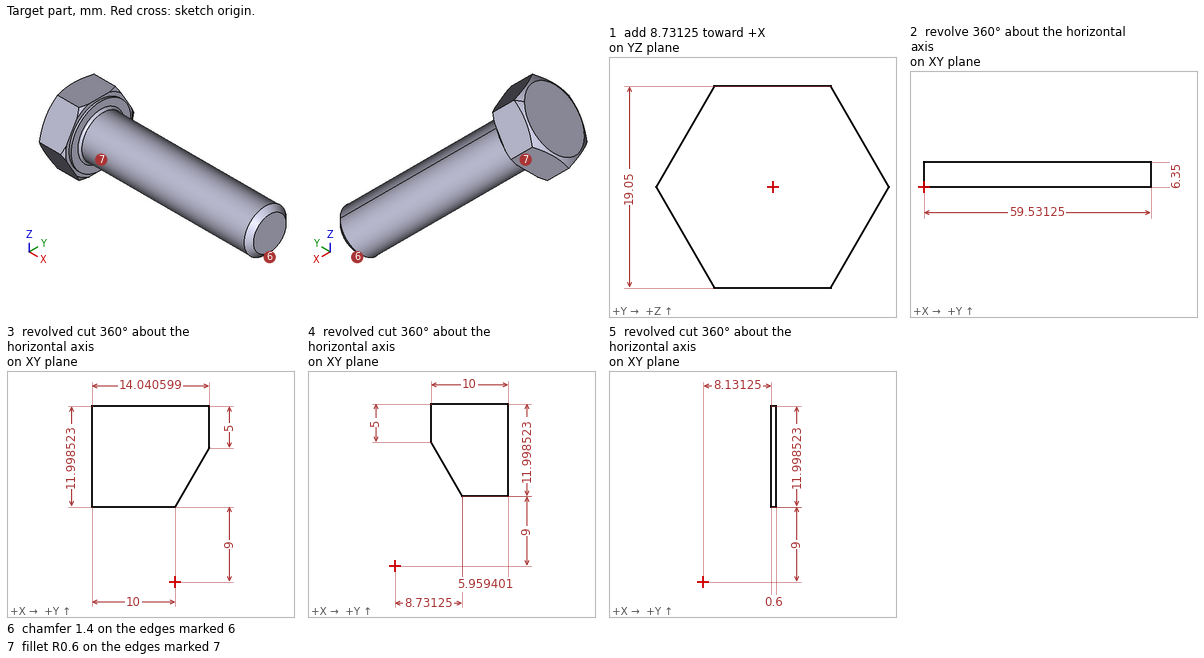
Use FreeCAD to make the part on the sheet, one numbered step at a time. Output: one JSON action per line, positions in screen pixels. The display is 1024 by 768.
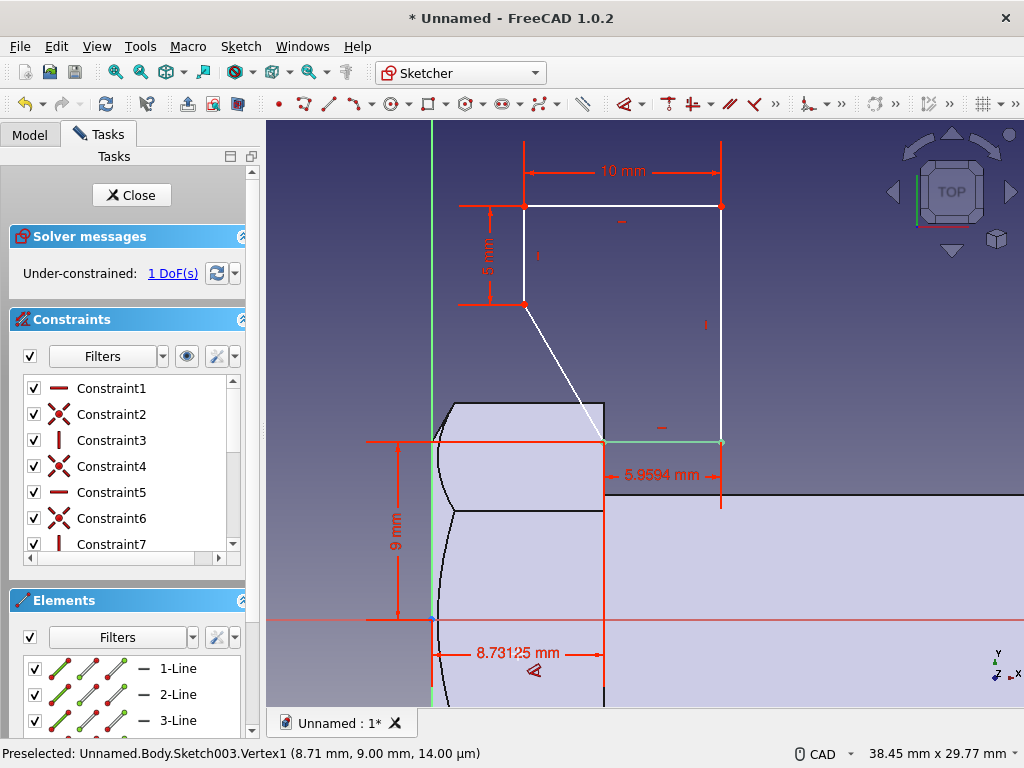
{"action": "left_click", "coordinate": [721, 372]}
{"action": "left_click", "coordinate": [755, 324]}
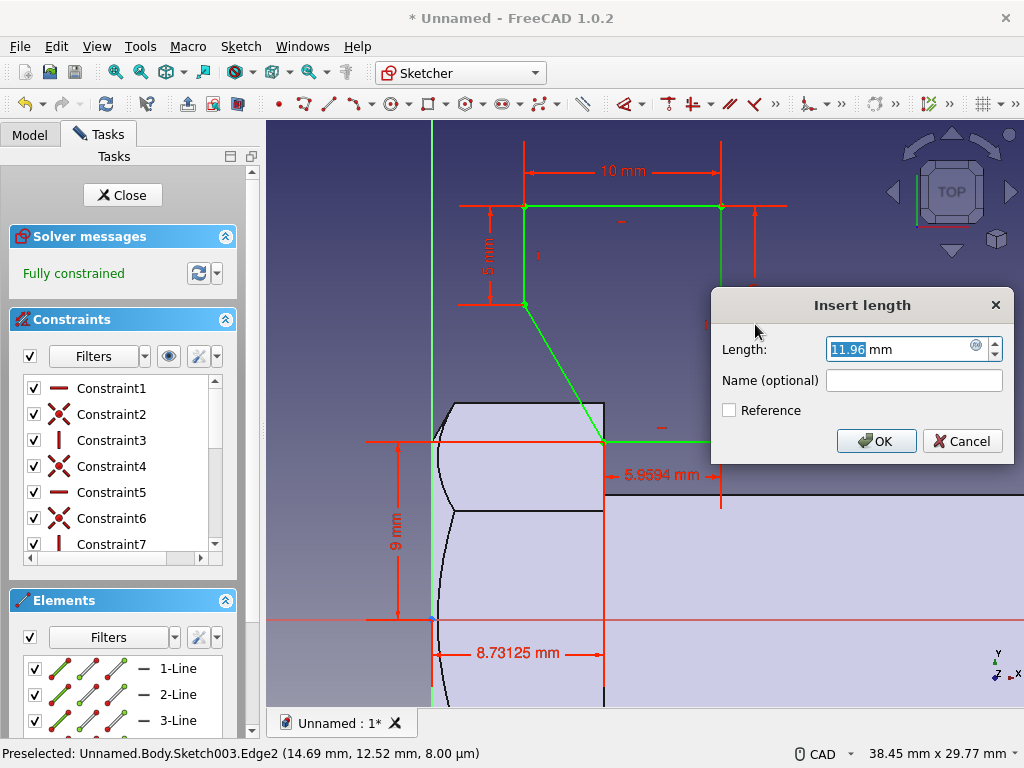
{"action": "type", "text": "11.998523"}
{"action": "key", "text": "Return"}
{"action": "key", "text": "Escape"}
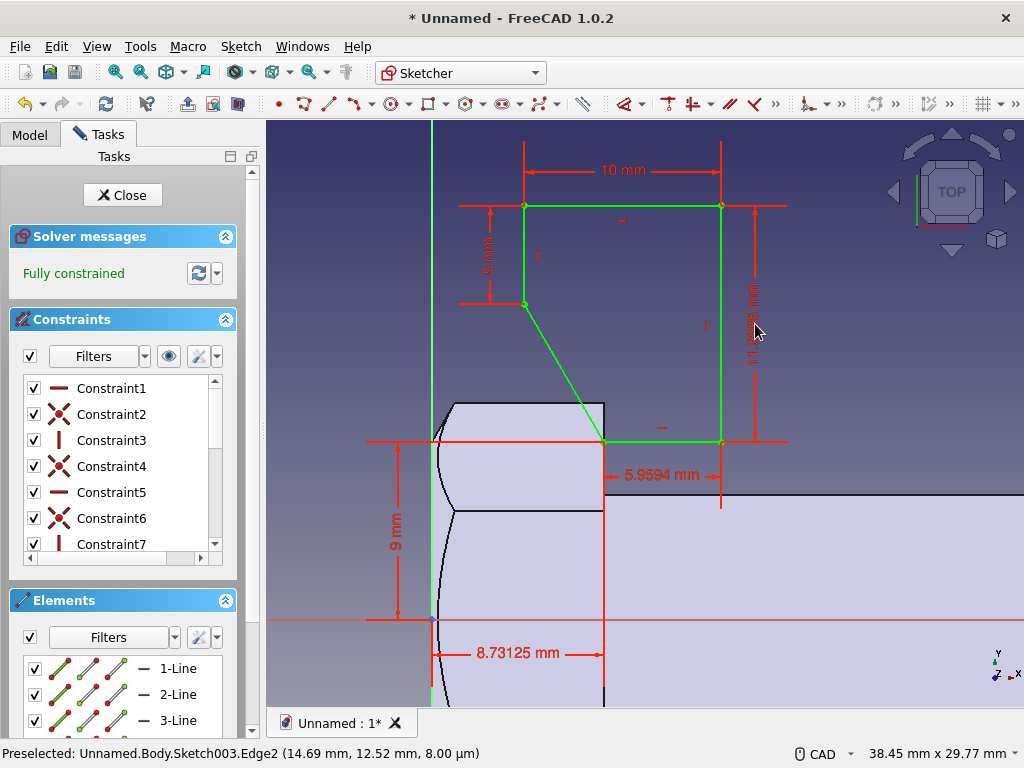
{"action": "left_click", "coordinate": [123, 195]}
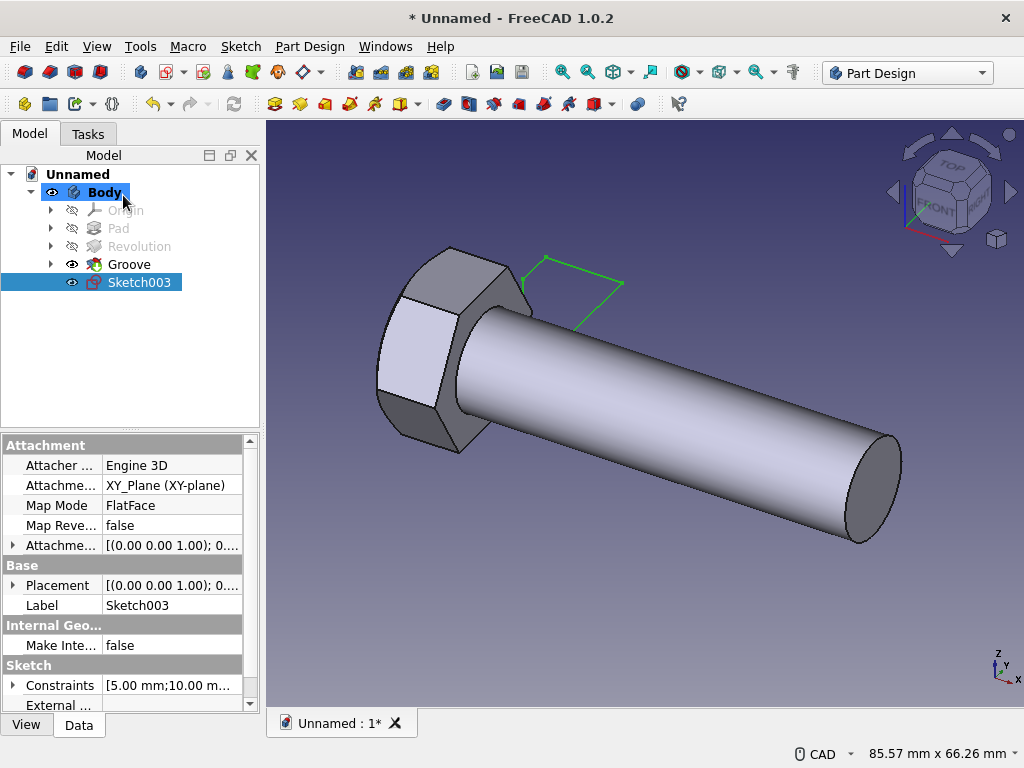
{"action": "left_click", "coordinate": [494, 104]}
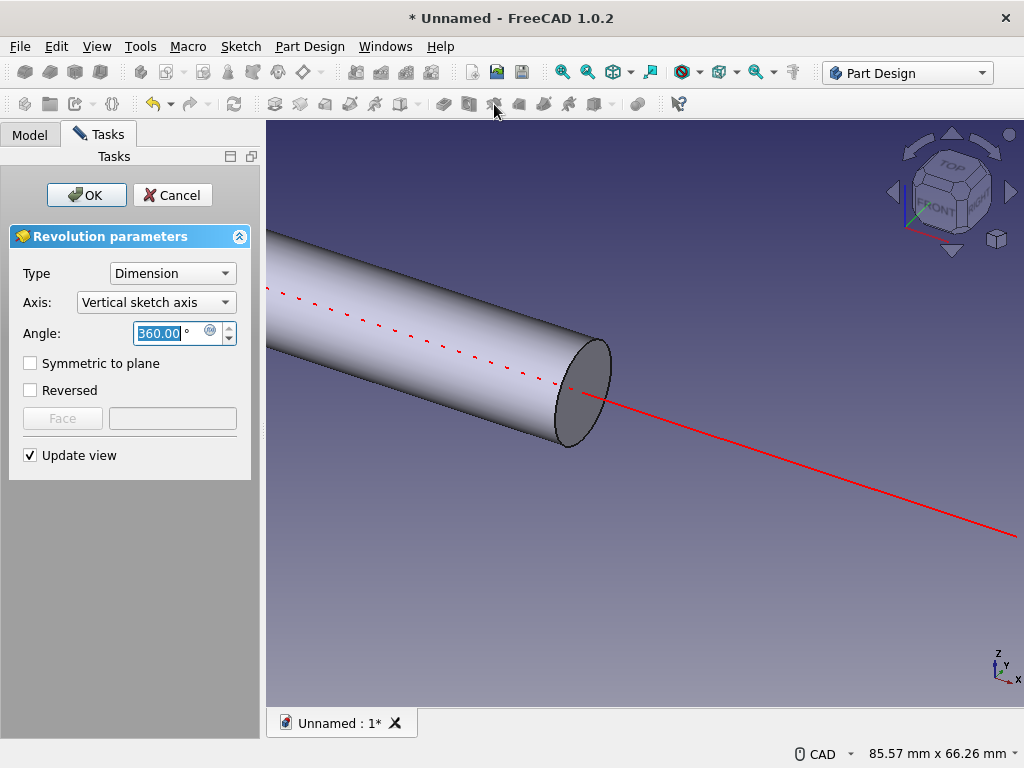
{"action": "left_click", "coordinate": [157, 302]}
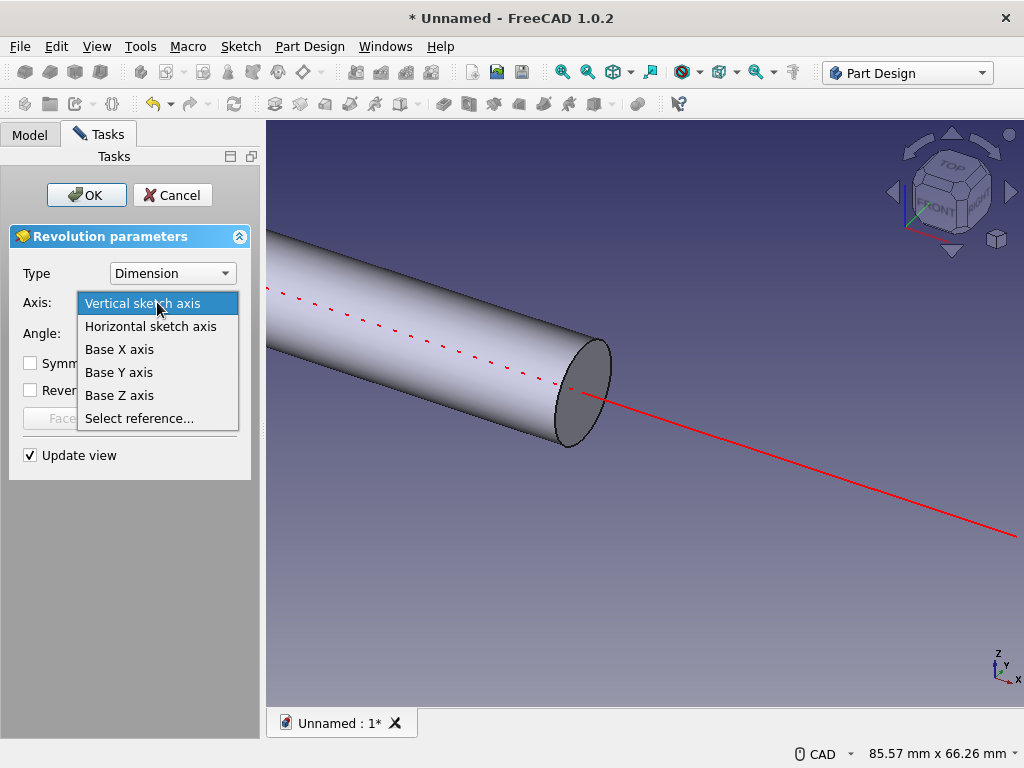
{"action": "left_click", "coordinate": [156, 326]}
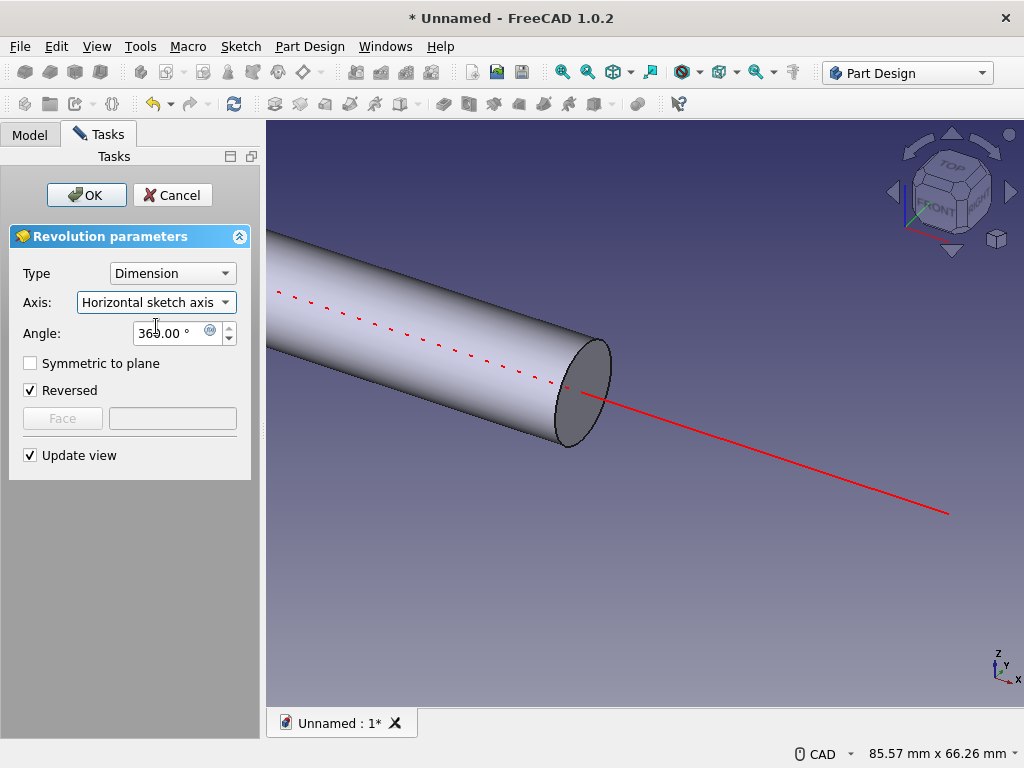
{"action": "left_click", "coordinate": [87, 195]}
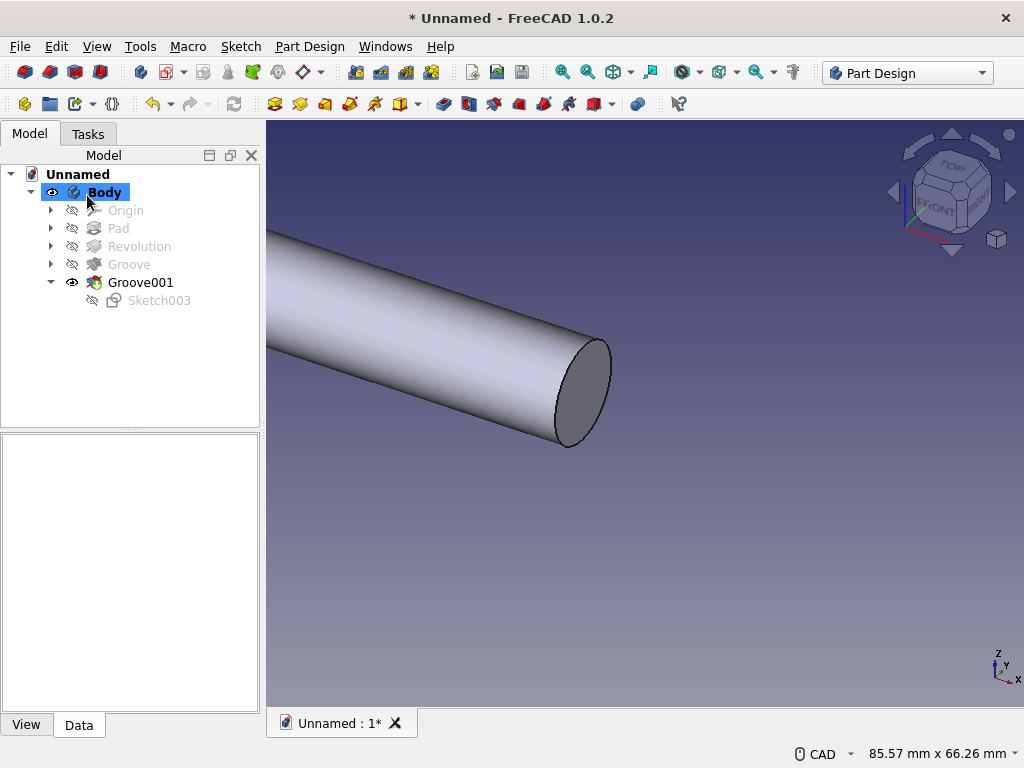
{"action": "left_click", "coordinate": [563, 72]}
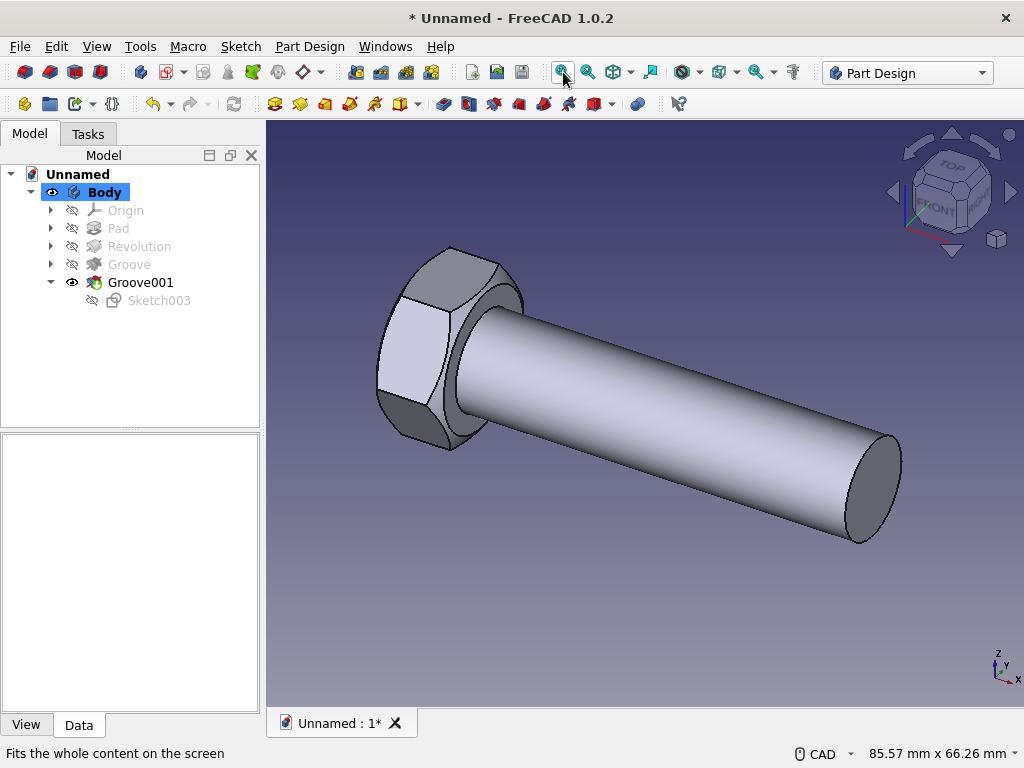
{"action": "left_click", "coordinate": [166, 72]}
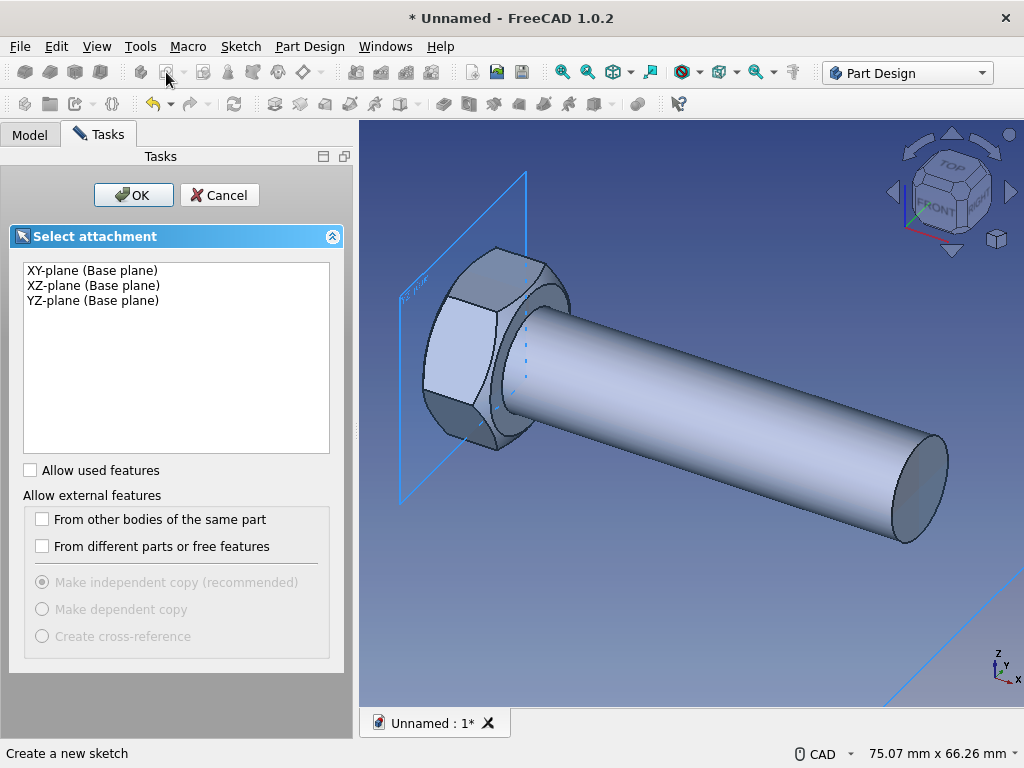
{"action": "left_click", "coordinate": [84, 270]}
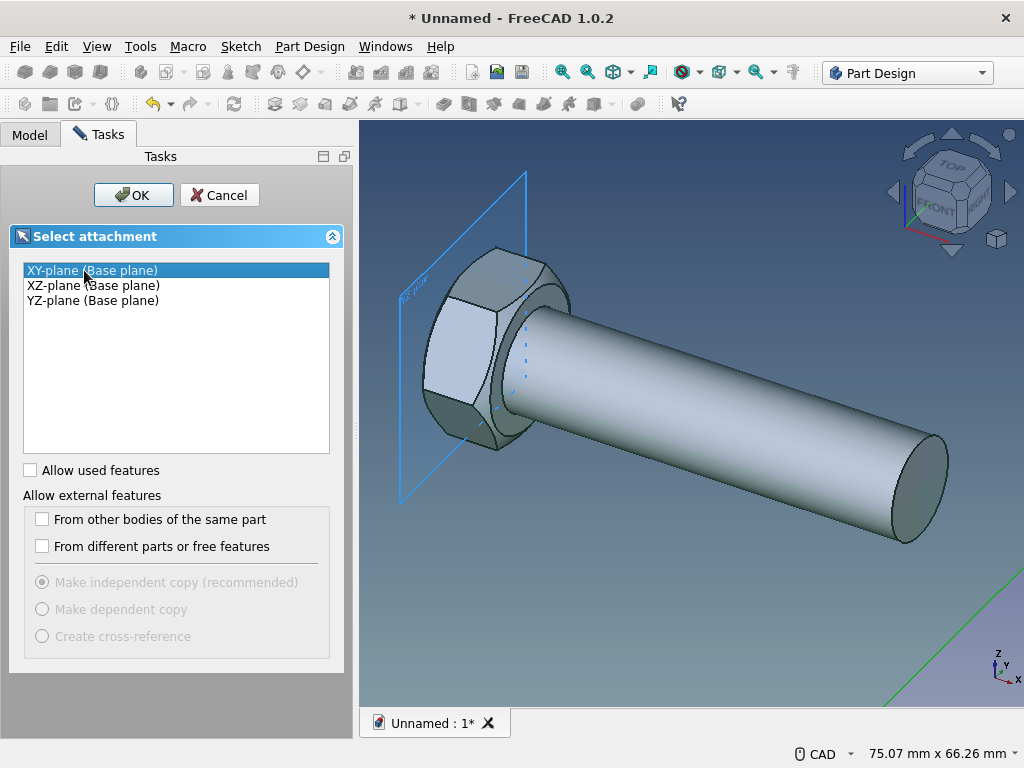
{"action": "left_click", "coordinate": [134, 195]}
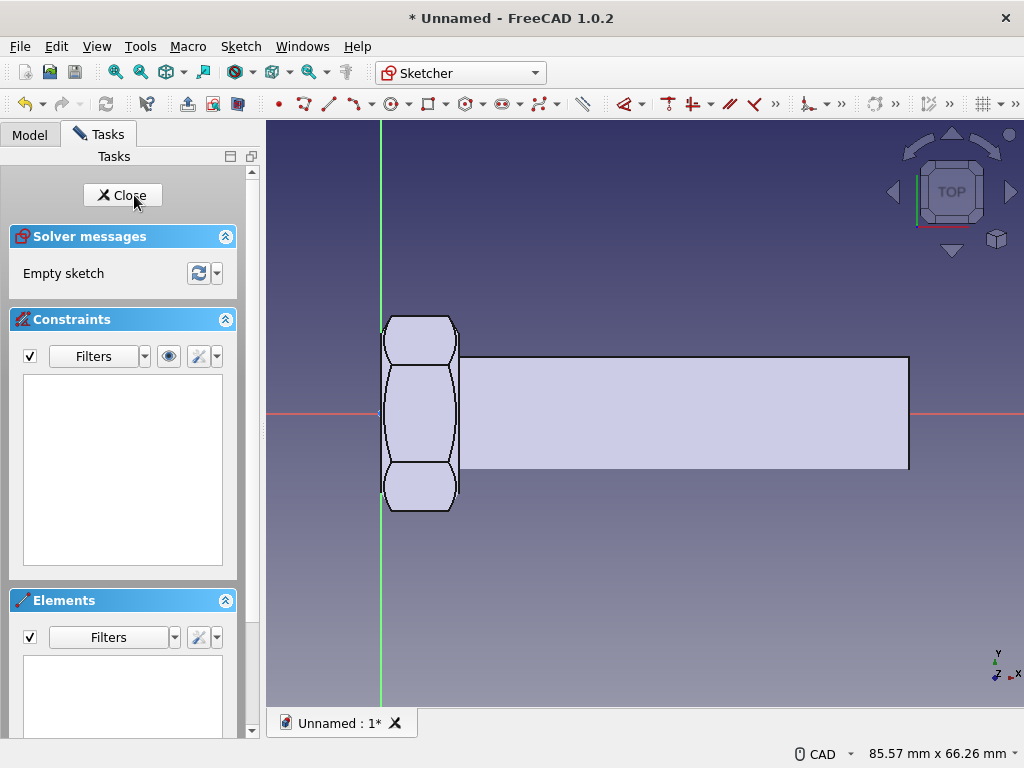
{"action": "left_click", "coordinate": [238, 104]}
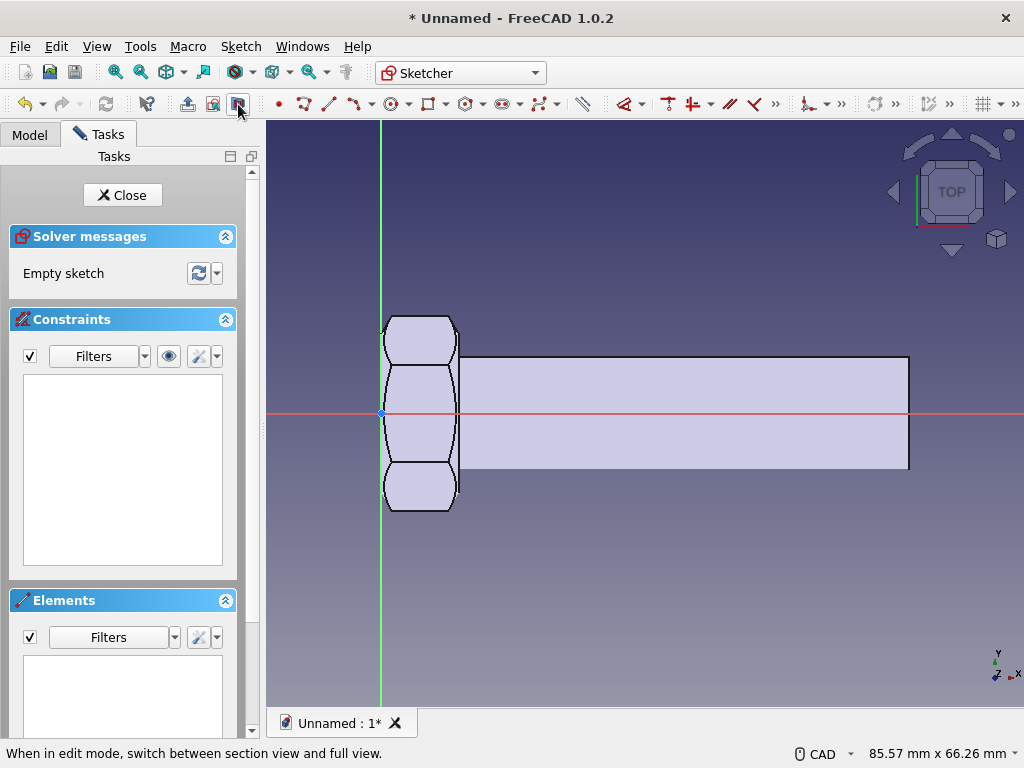
{"action": "scroll", "coordinate": [294, 245], "scroll_direction": "up", "scroll_amount": 4}